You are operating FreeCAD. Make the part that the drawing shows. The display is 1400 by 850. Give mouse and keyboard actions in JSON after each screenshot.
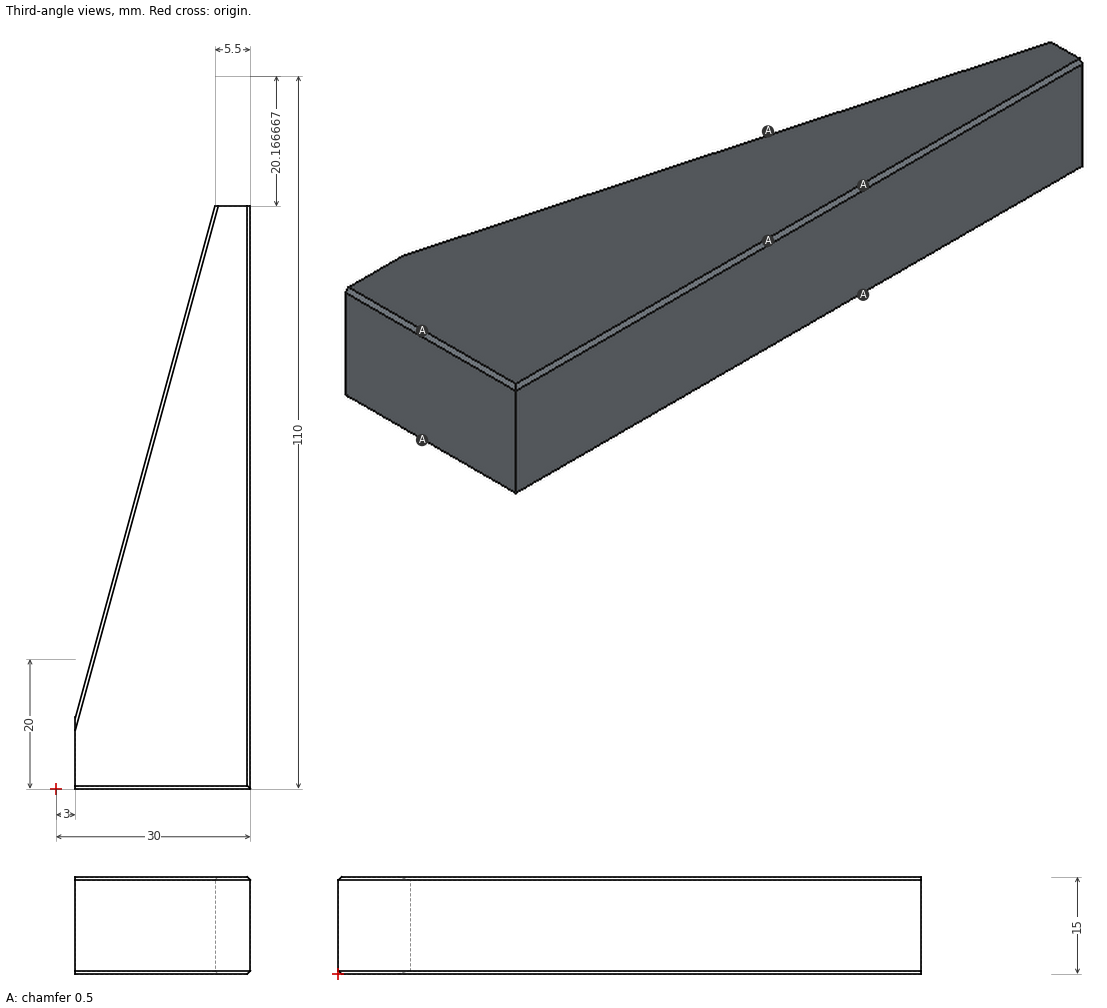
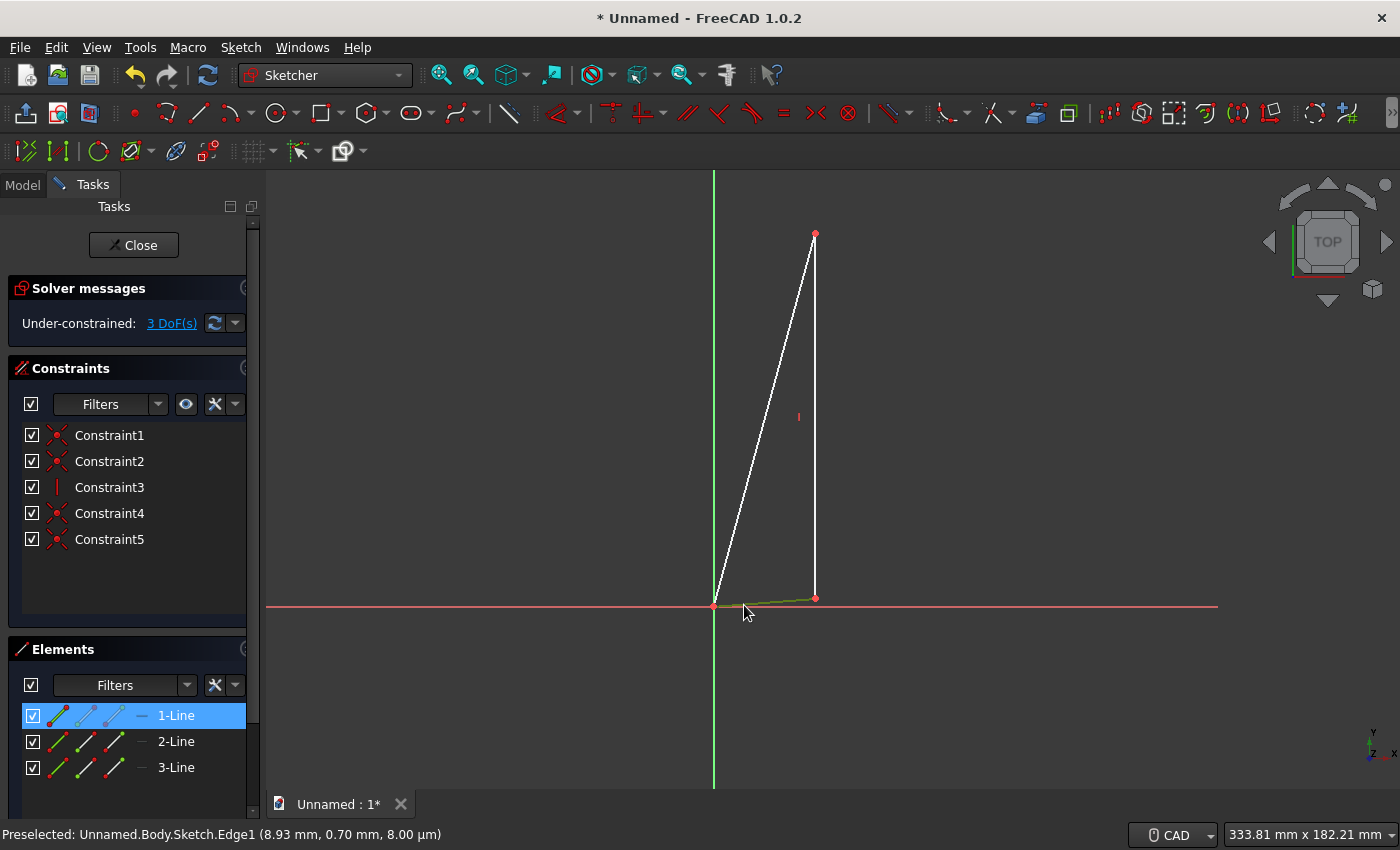
{"action": "key", "text": "h"}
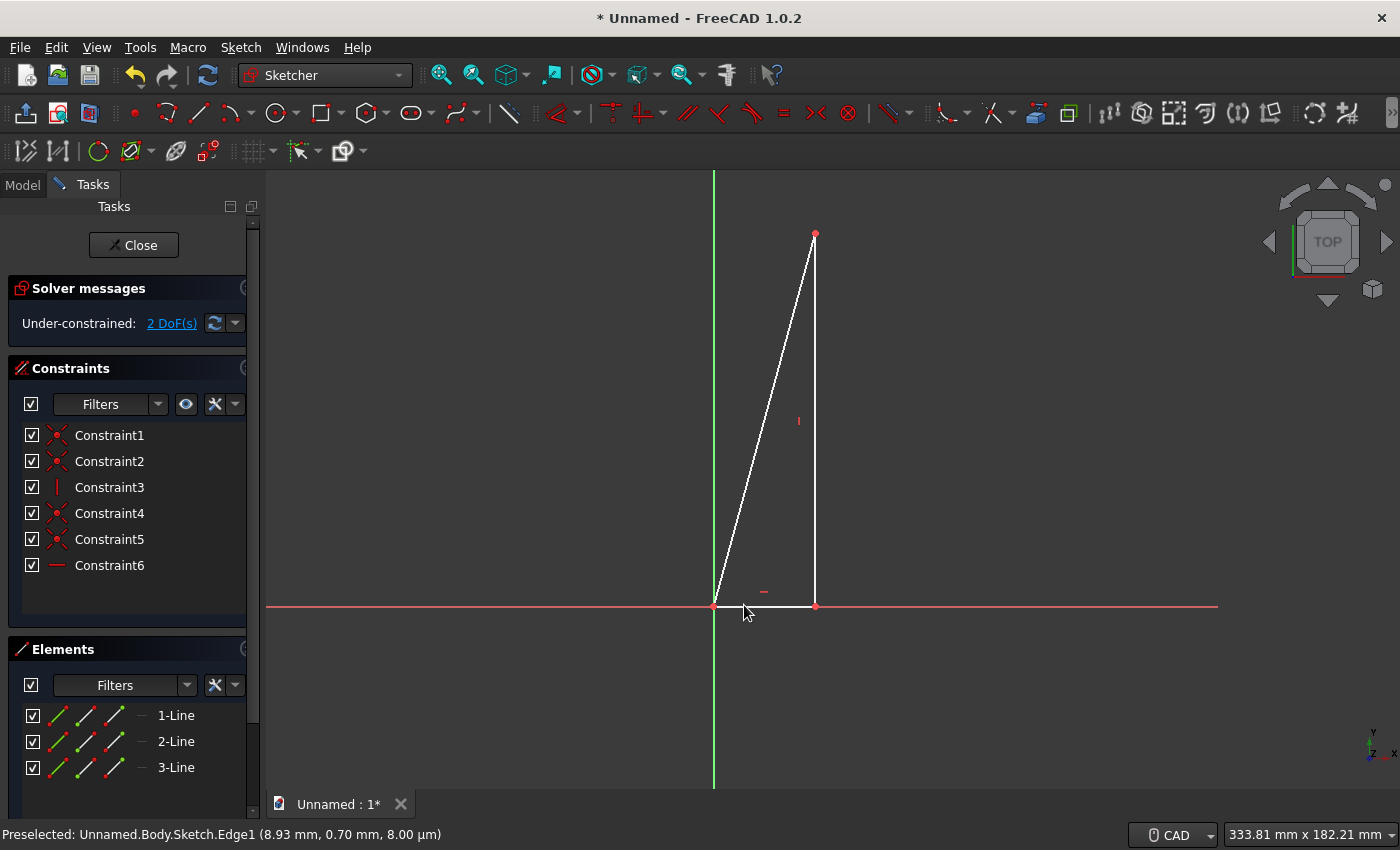
{"action": "left_click", "coordinate": [556, 114]}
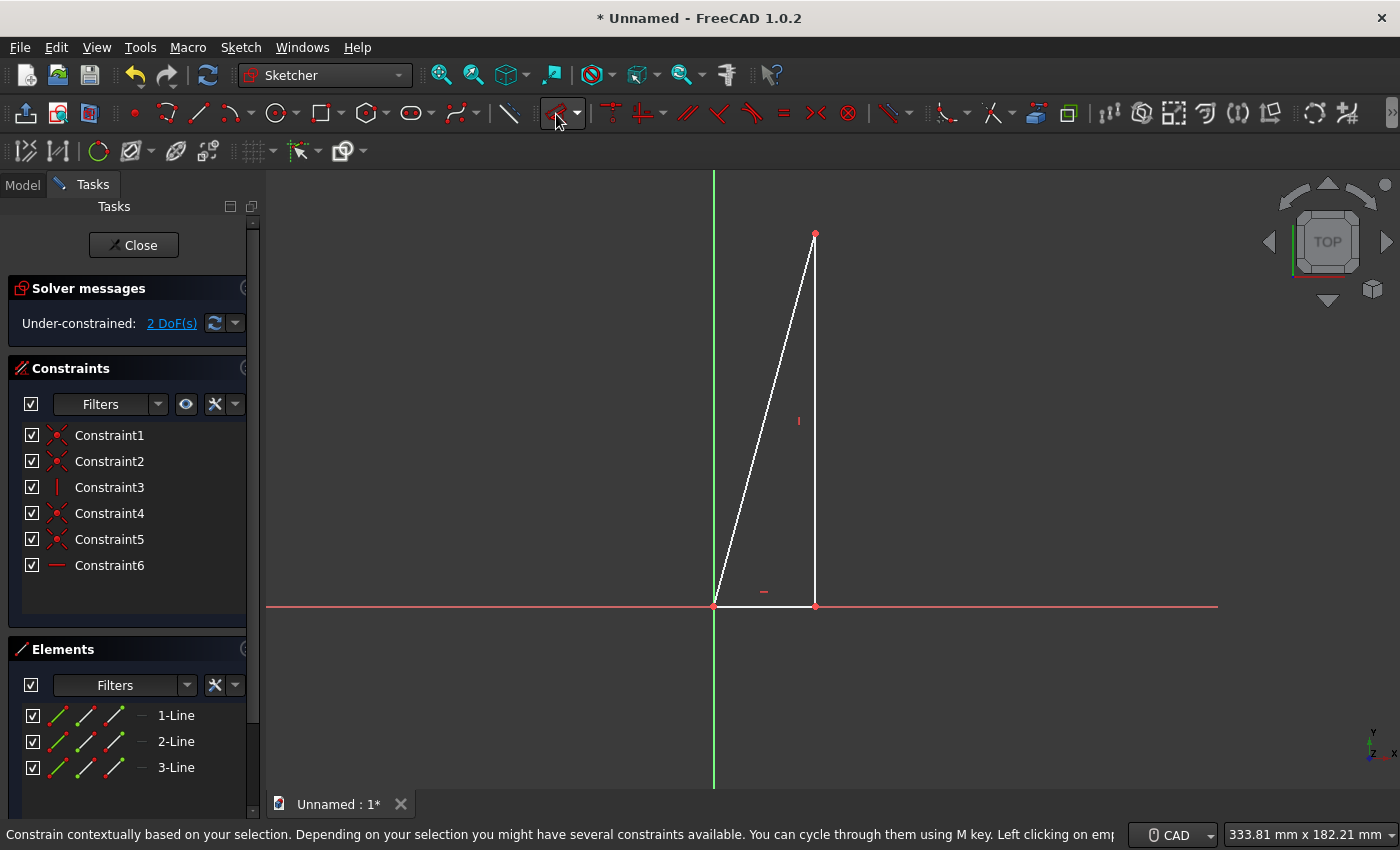
{"action": "left_click", "coordinate": [744, 607]}
{"action": "left_click", "coordinate": [764, 641]}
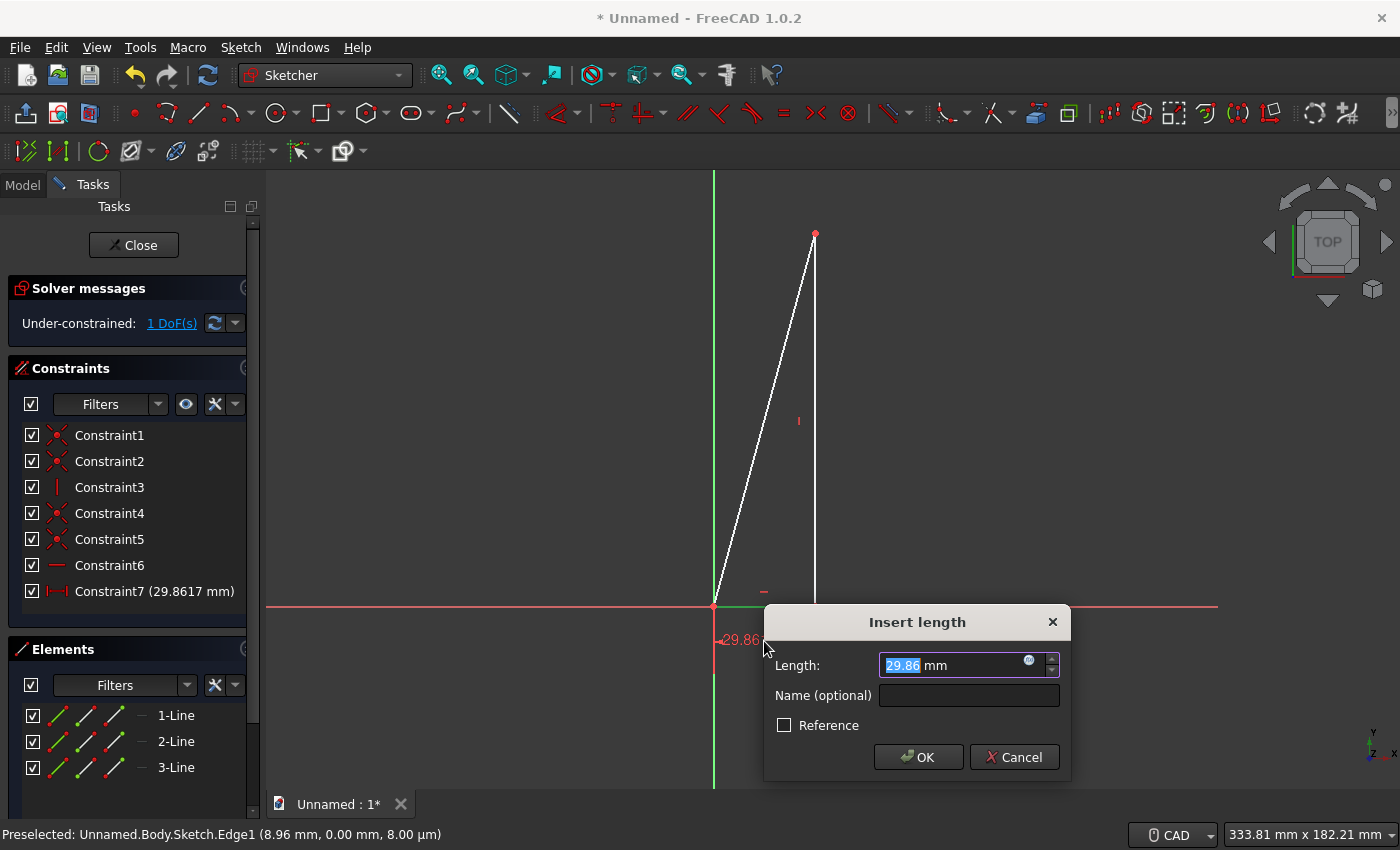
{"action": "type", "text": "30"}
{"action": "key", "text": "Return"}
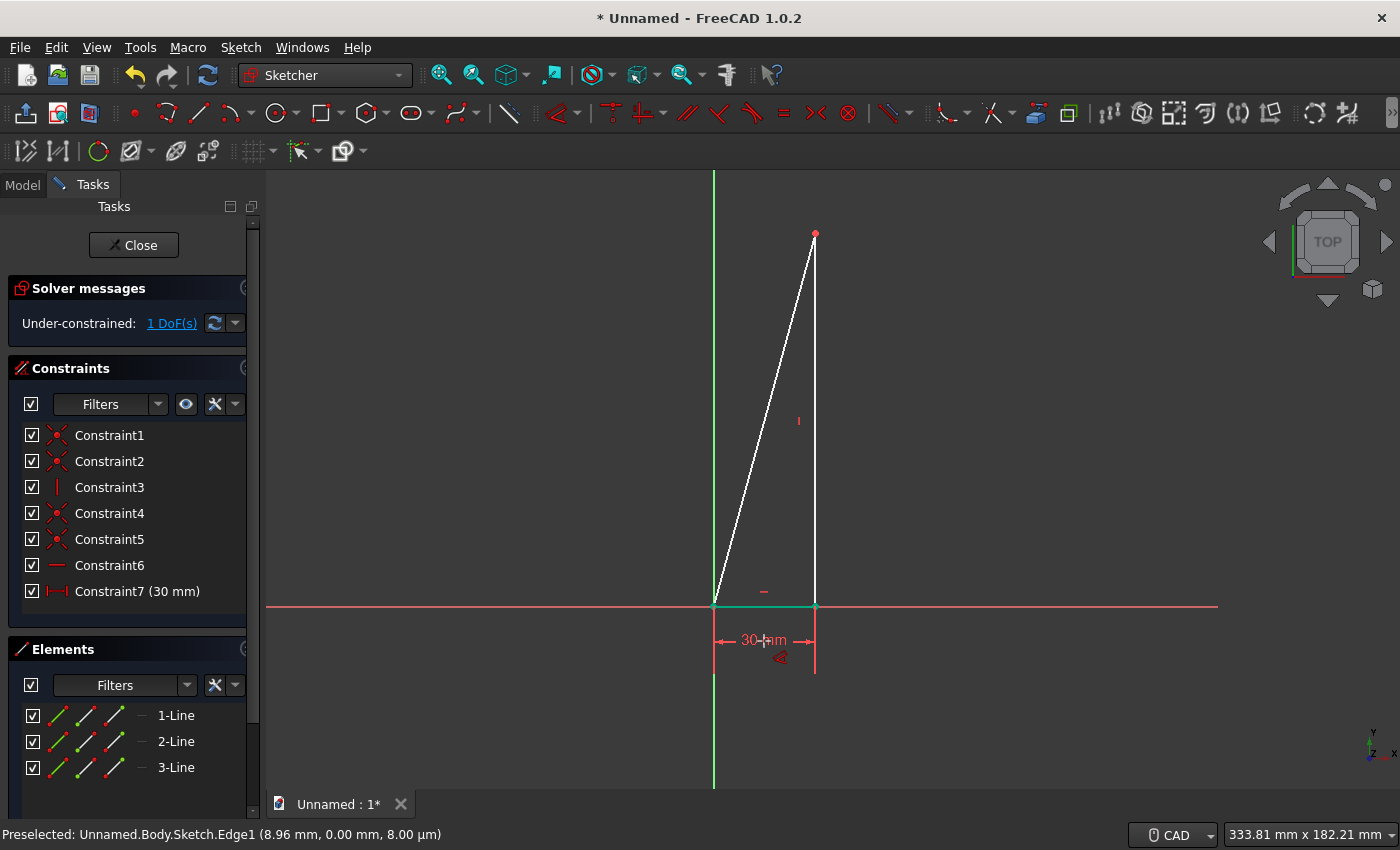
{"action": "left_click", "coordinate": [815, 495]}
{"action": "left_click", "coordinate": [849, 420]}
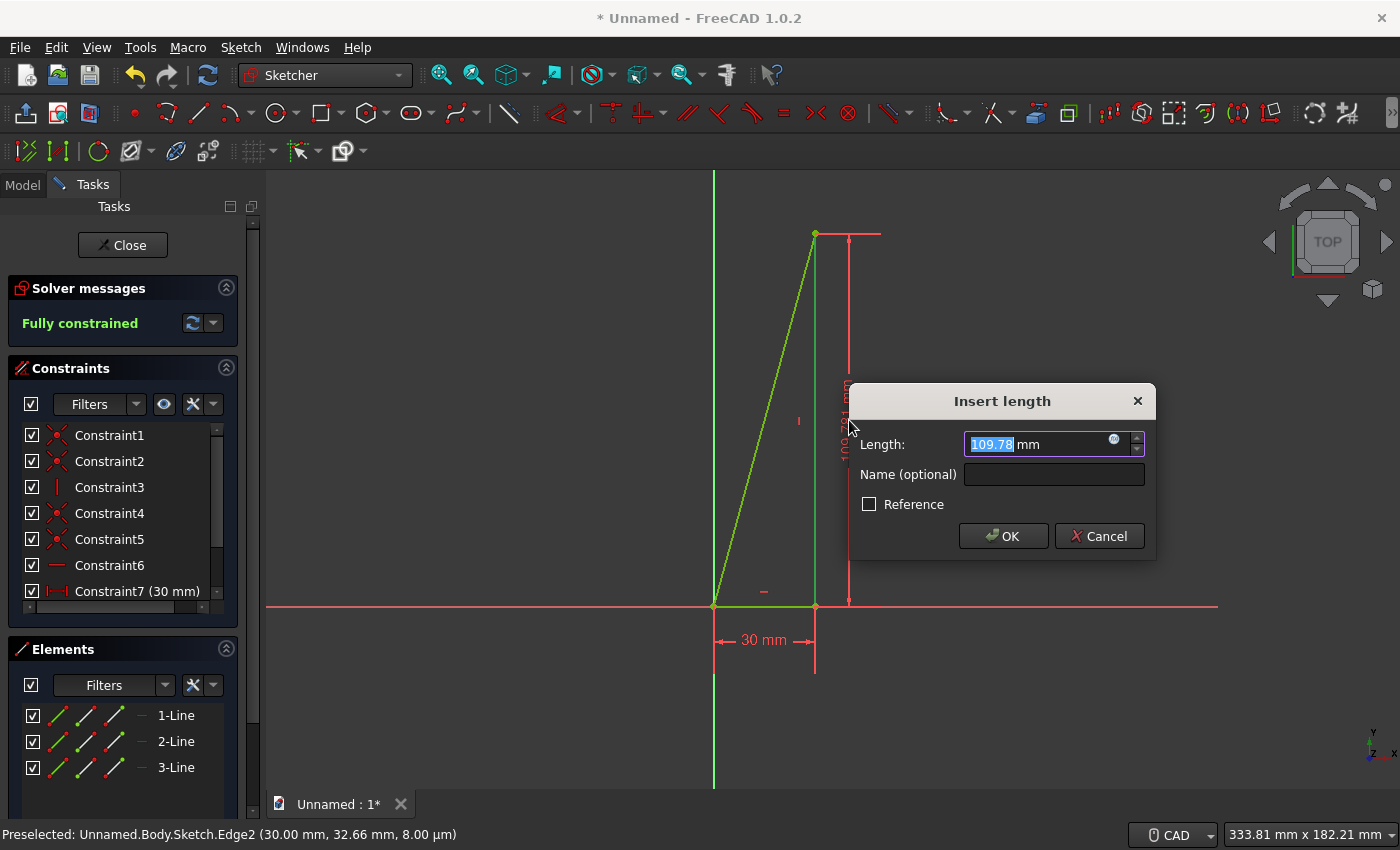
{"action": "type", "text": "110"}
{"action": "key", "text": "Return"}
{"action": "key", "text": "Escape"}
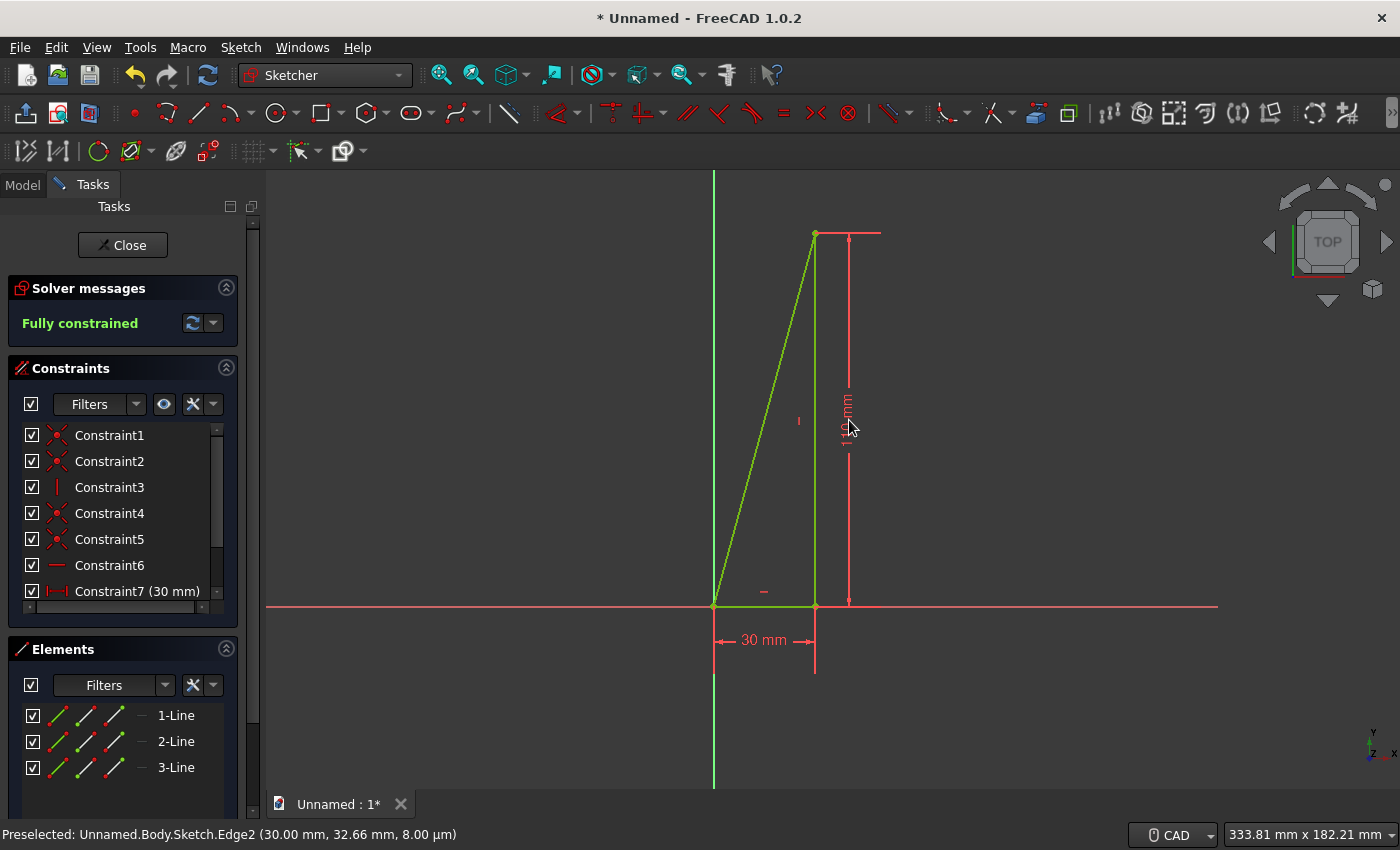
{"action": "left_click", "coordinate": [123, 245]}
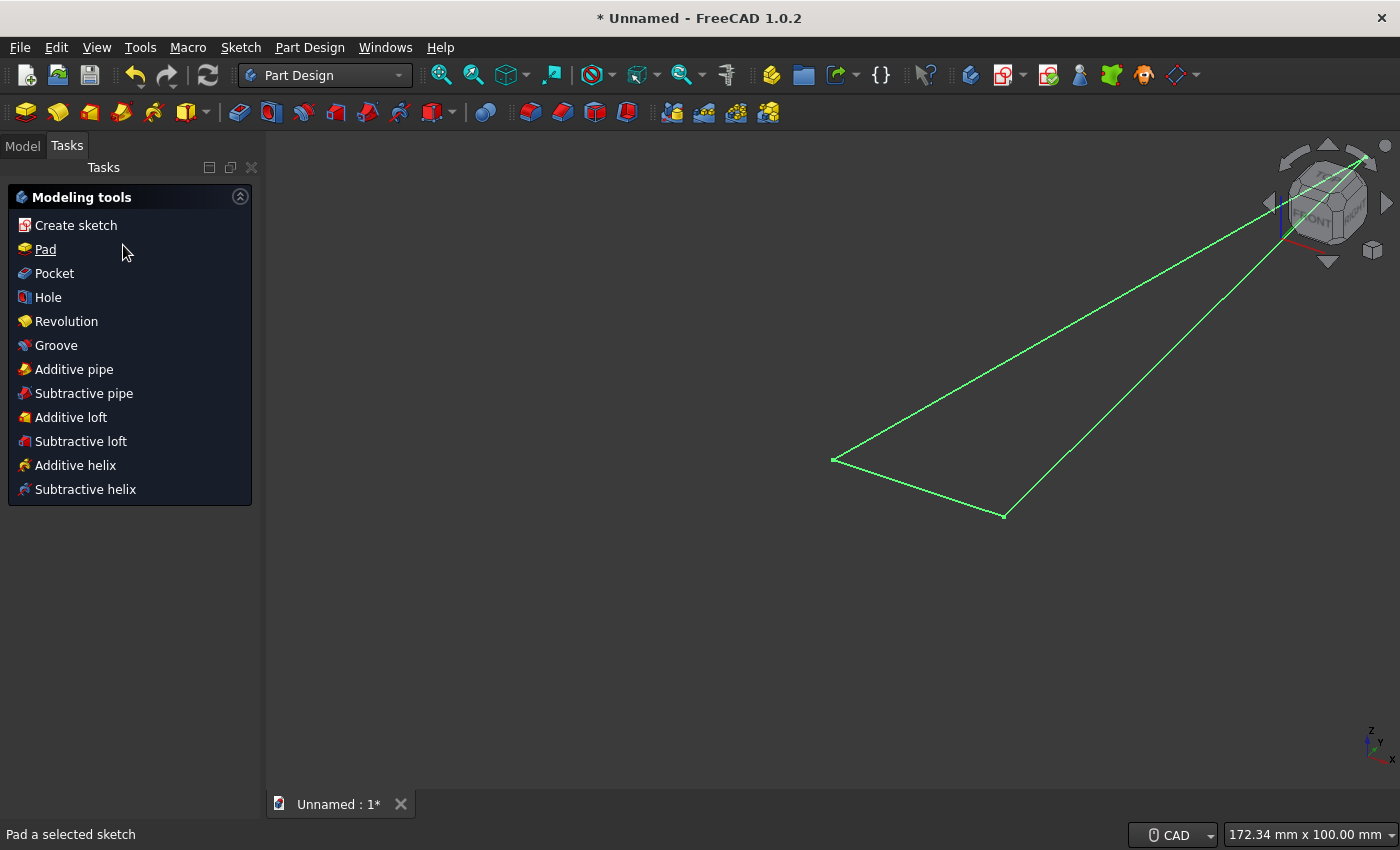
{"action": "left_click", "coordinate": [26, 112]}